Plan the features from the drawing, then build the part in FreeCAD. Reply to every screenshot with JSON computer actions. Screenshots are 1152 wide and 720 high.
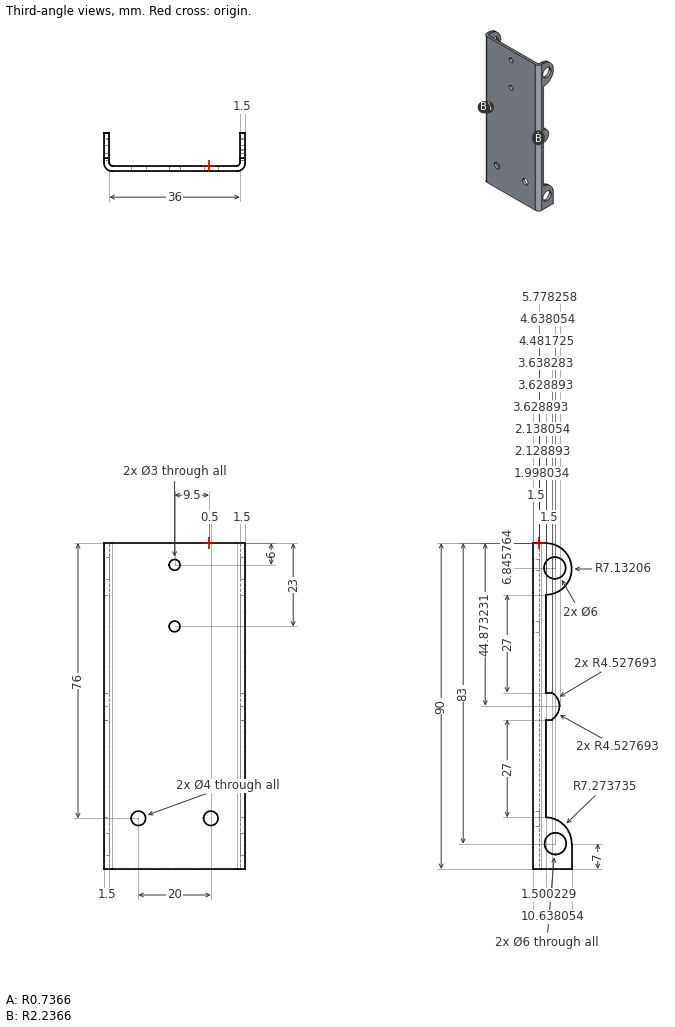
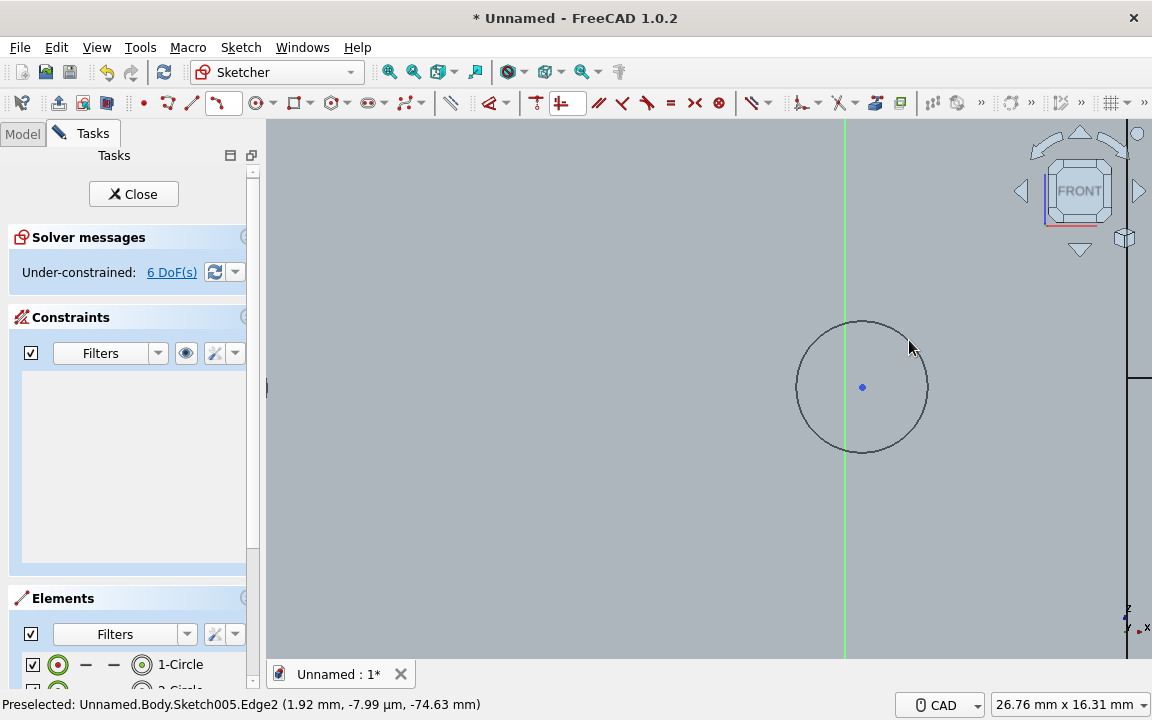
{"action": "scroll", "coordinate": [864, 394], "scroll_direction": "down", "scroll_amount": 2}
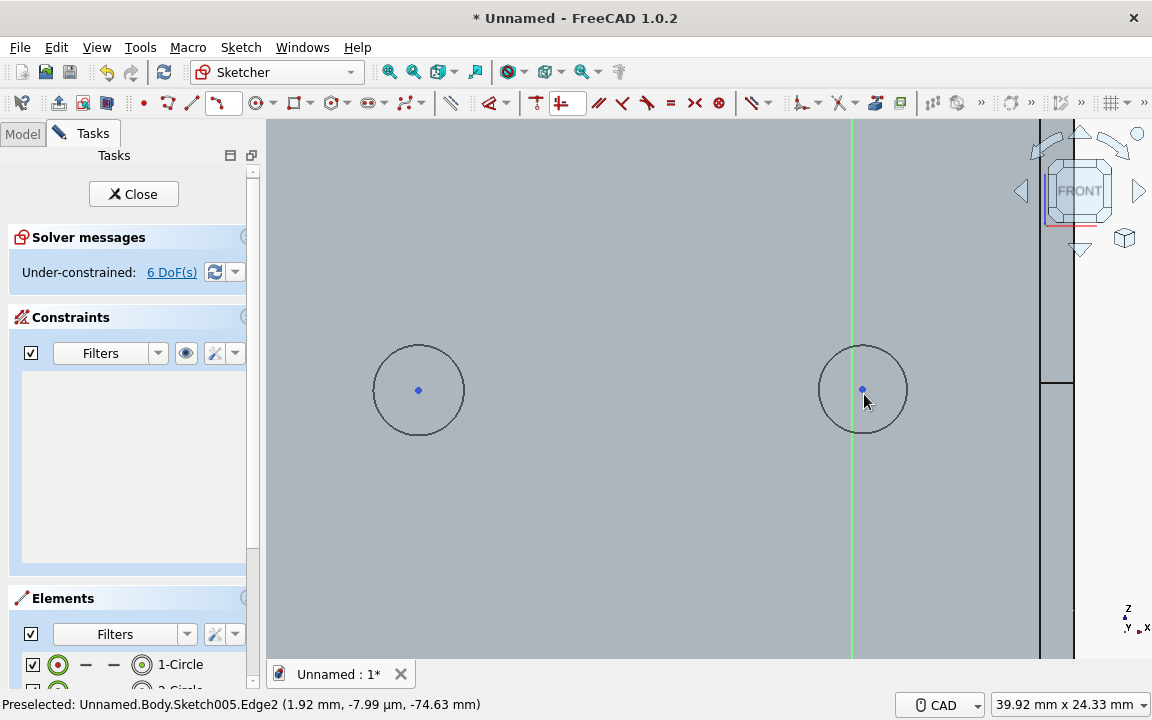
{"action": "left_click", "coordinate": [451, 358]}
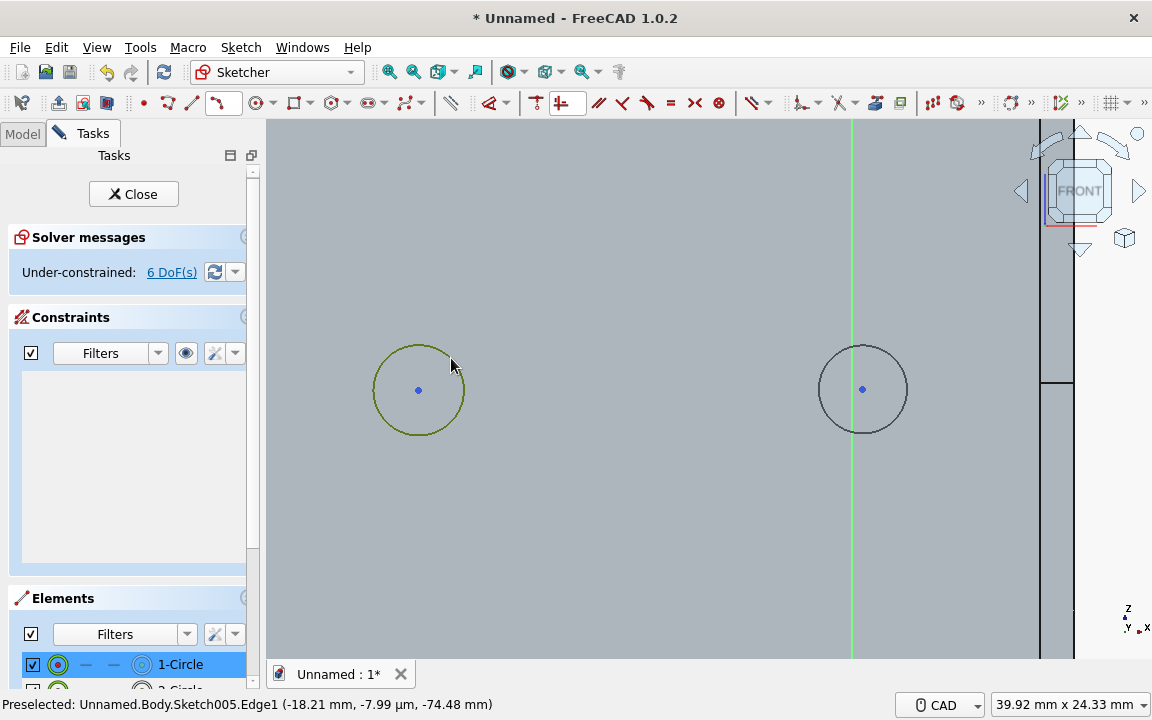
{"action": "left_click", "coordinate": [894, 358]}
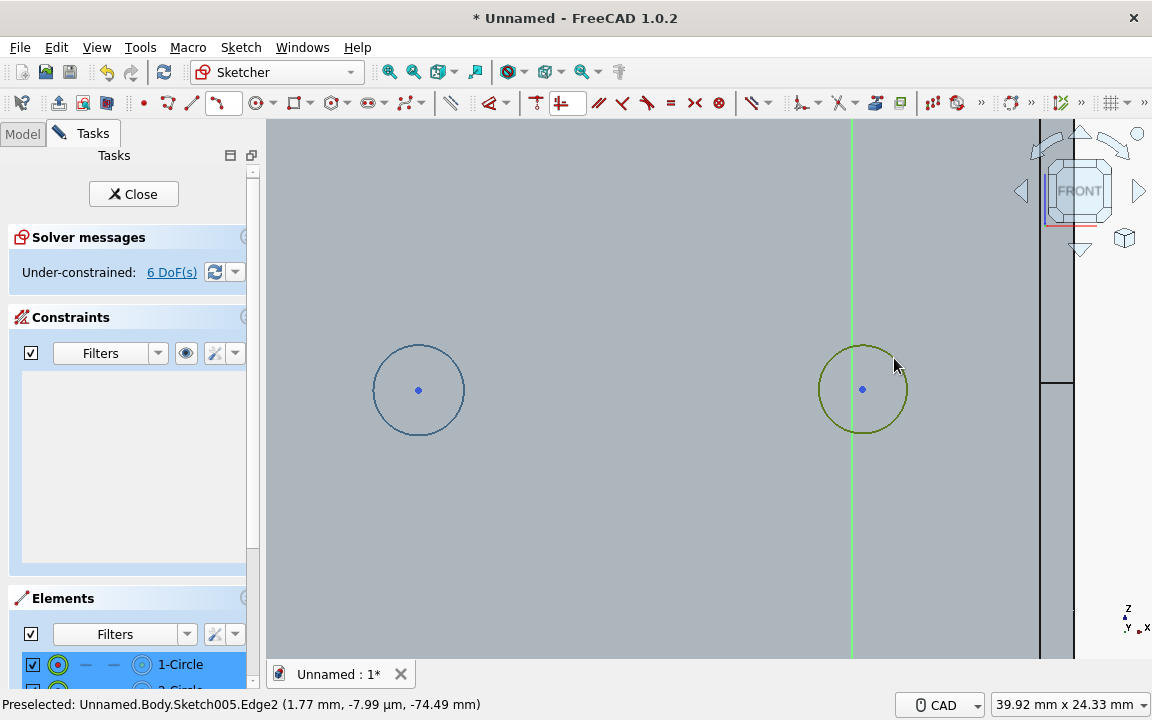
{"action": "key", "text": "e"}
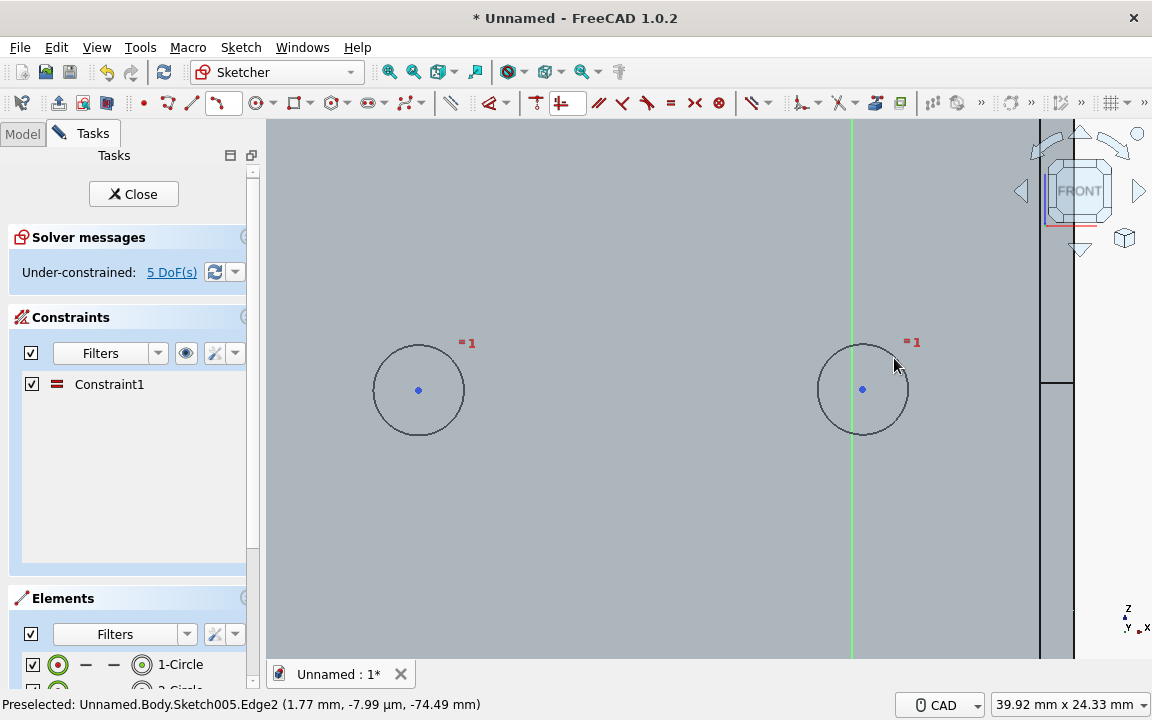
{"action": "left_click", "coordinate": [419, 390]}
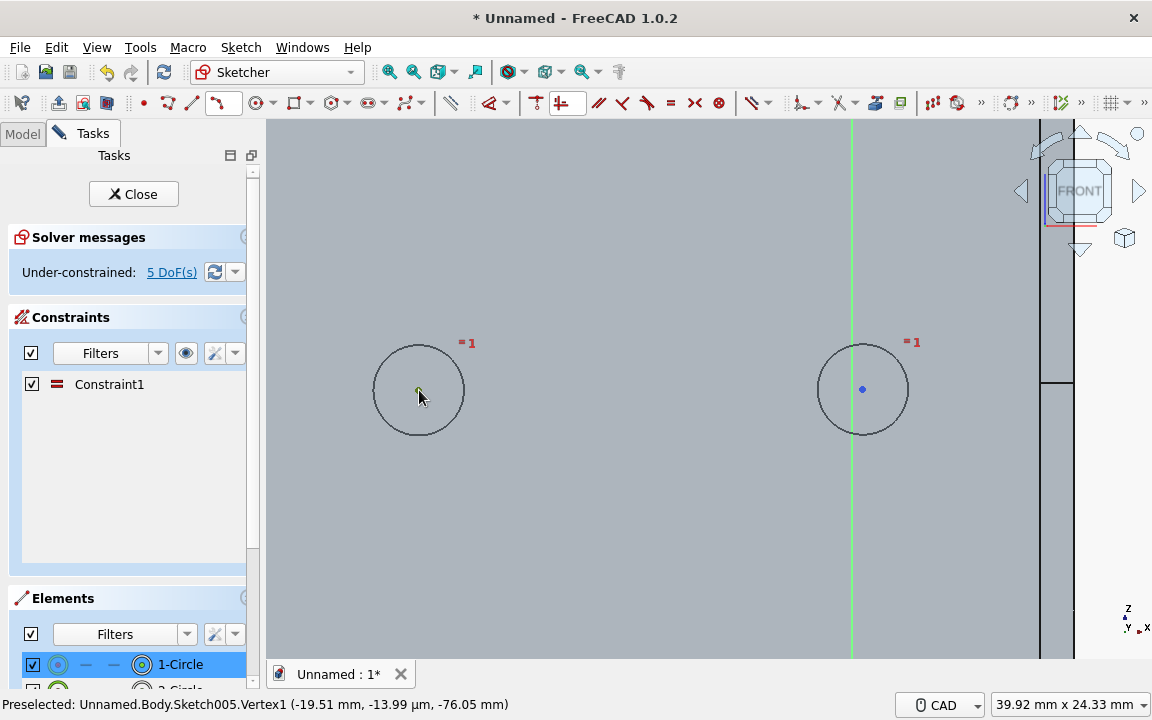
{"action": "left_click", "coordinate": [863, 389]}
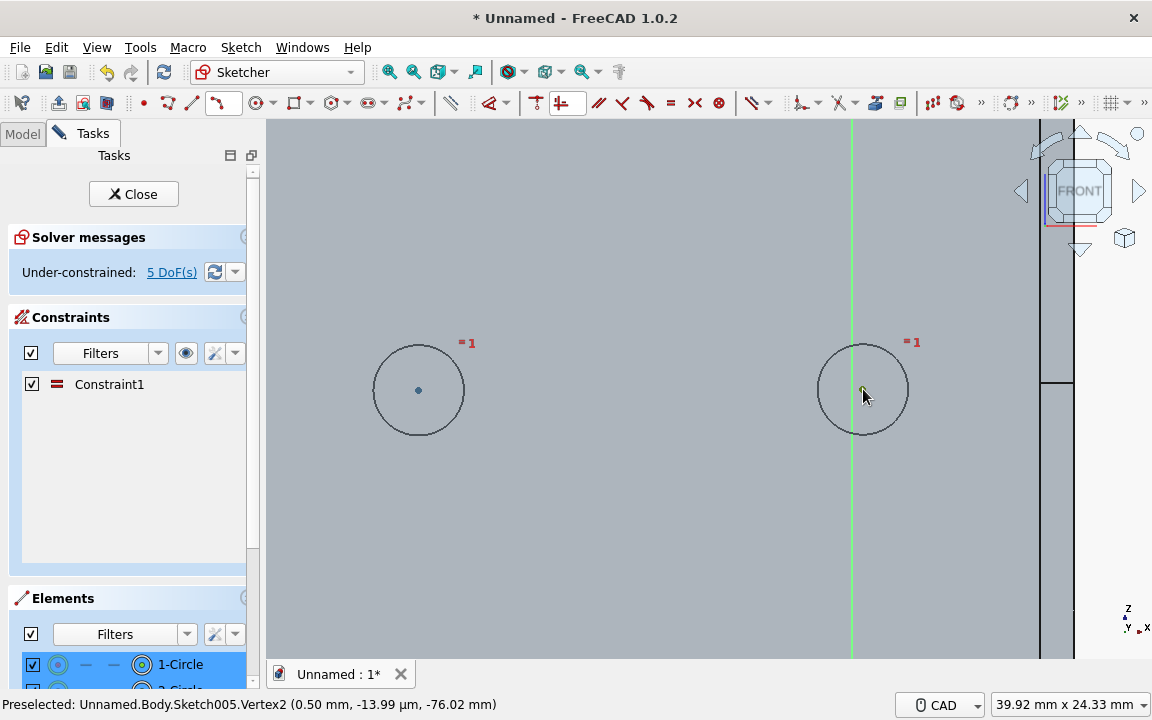
{"action": "key", "text": "h"}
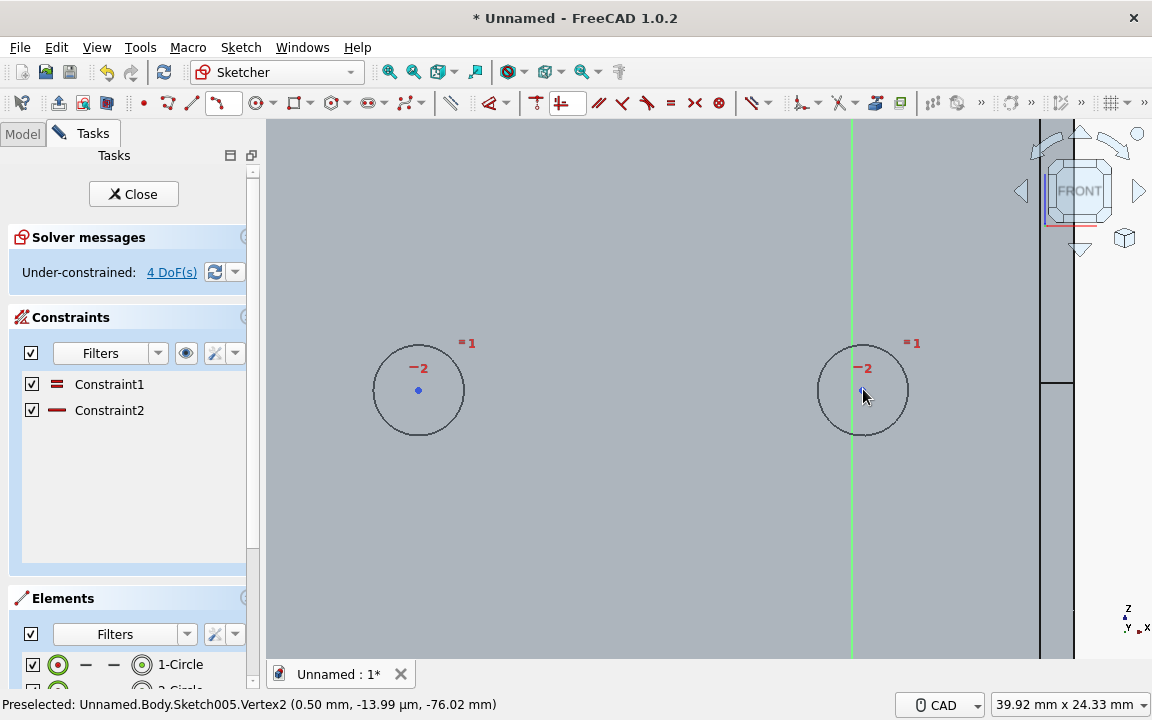
{"action": "key", "text": "d"}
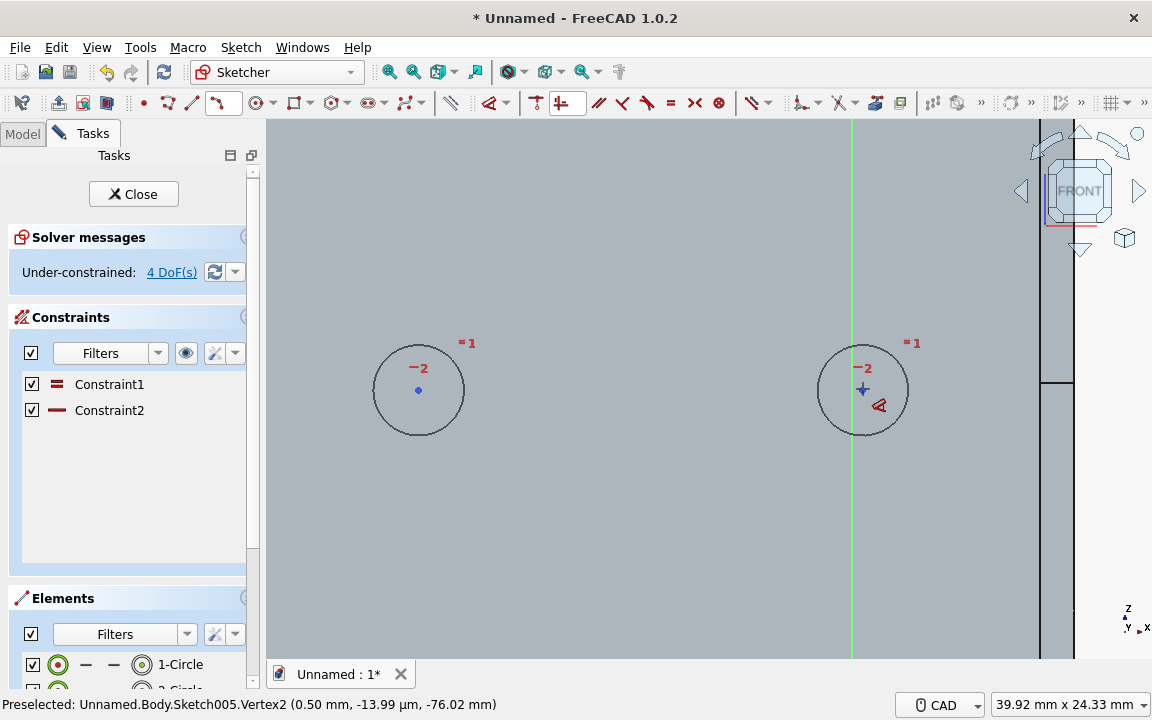
{"action": "left_click", "coordinate": [451, 358]}
{"action": "left_click", "coordinate": [474, 335]}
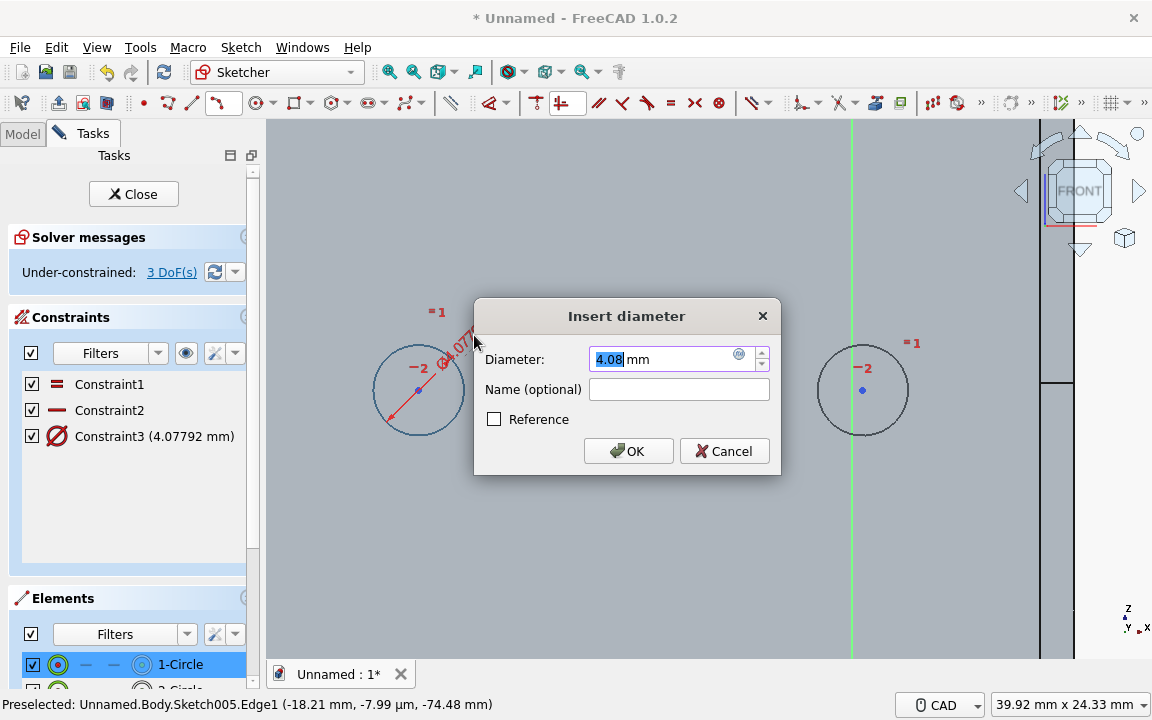
{"action": "type", "text": "4"}
{"action": "key", "text": "Return"}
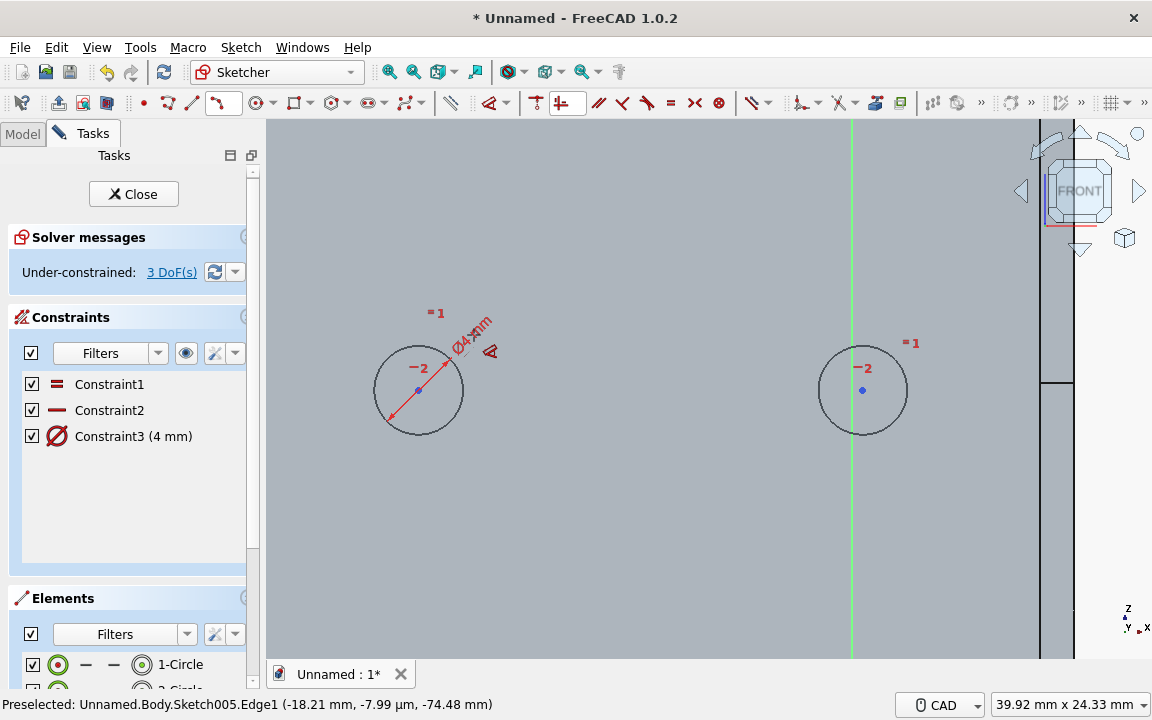
{"action": "left_click", "coordinate": [419, 390]}
{"action": "left_click", "coordinate": [385, 269]}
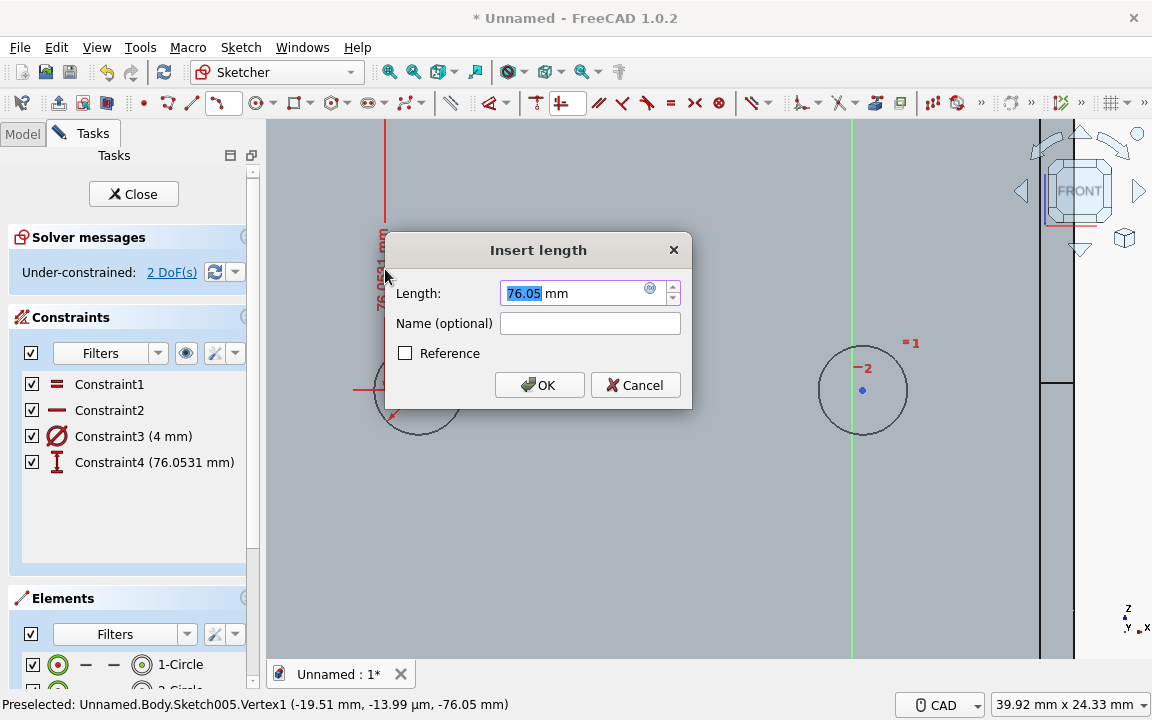
{"action": "type", "text": "76"}
{"action": "key", "text": "Return"}